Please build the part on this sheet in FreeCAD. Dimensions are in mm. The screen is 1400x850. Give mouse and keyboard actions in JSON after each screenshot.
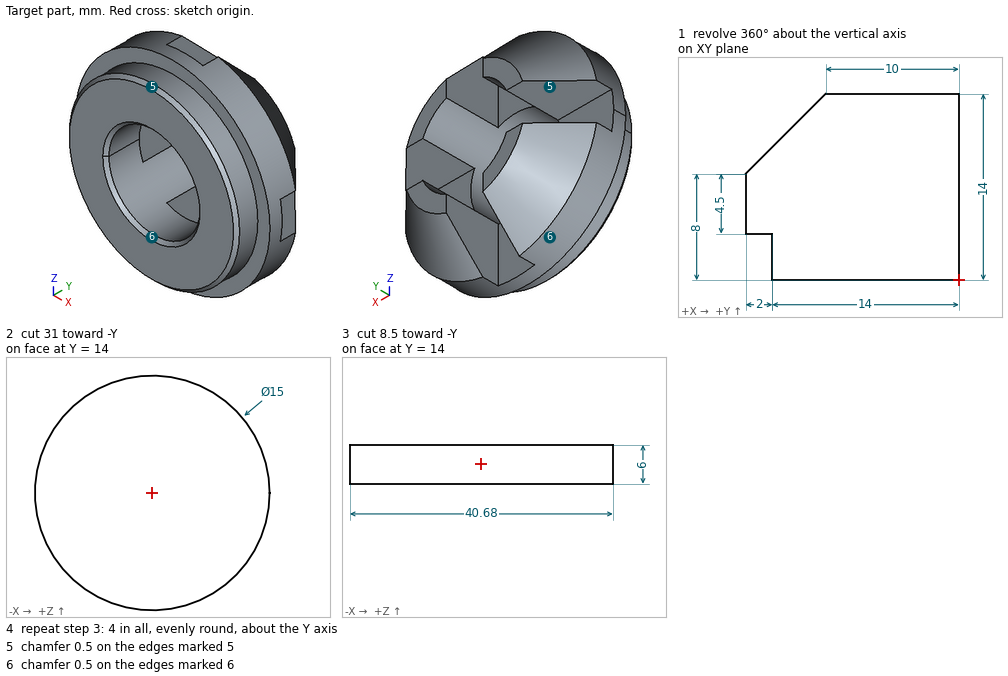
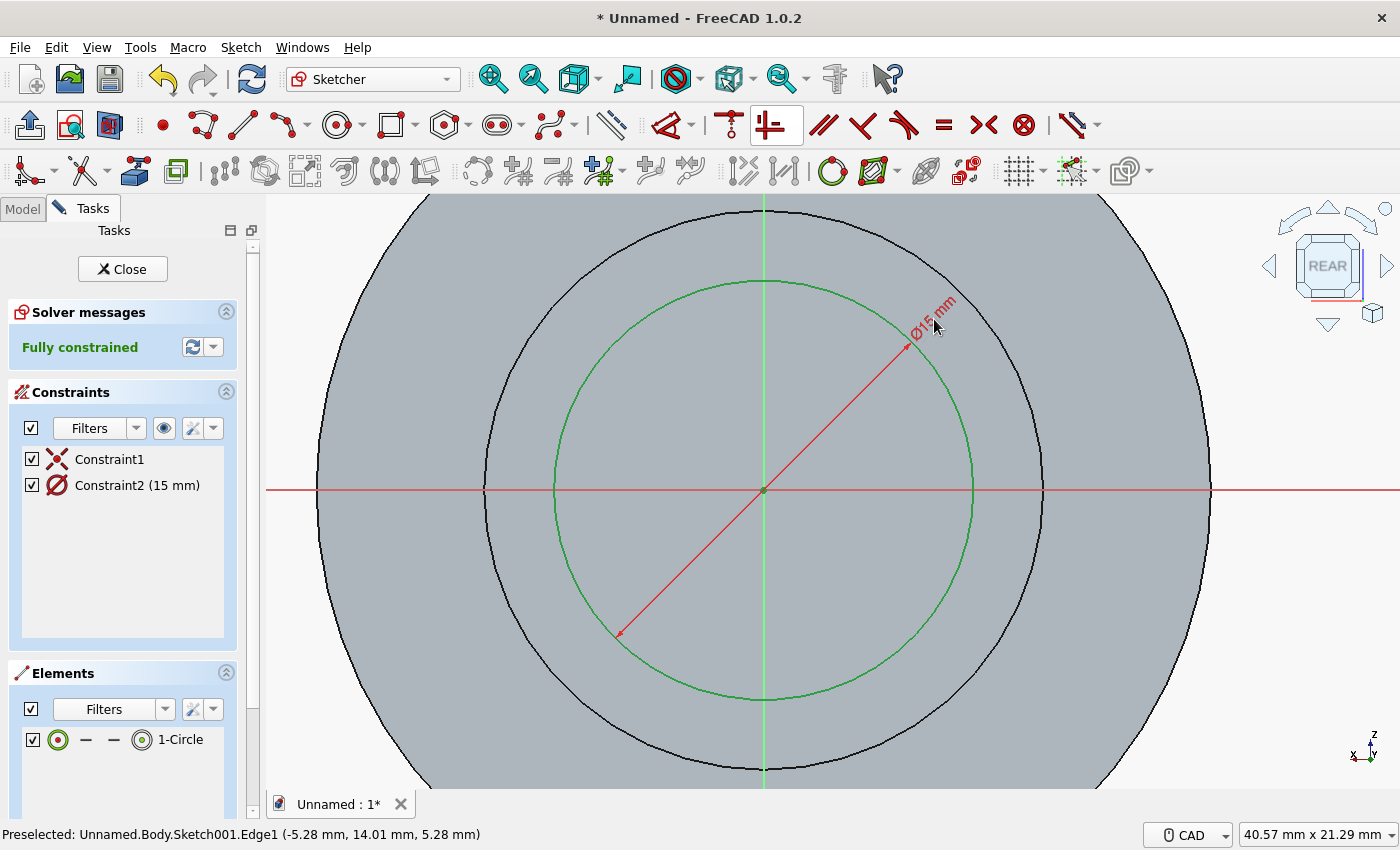
{"action": "left_click", "coordinate": [123, 269]}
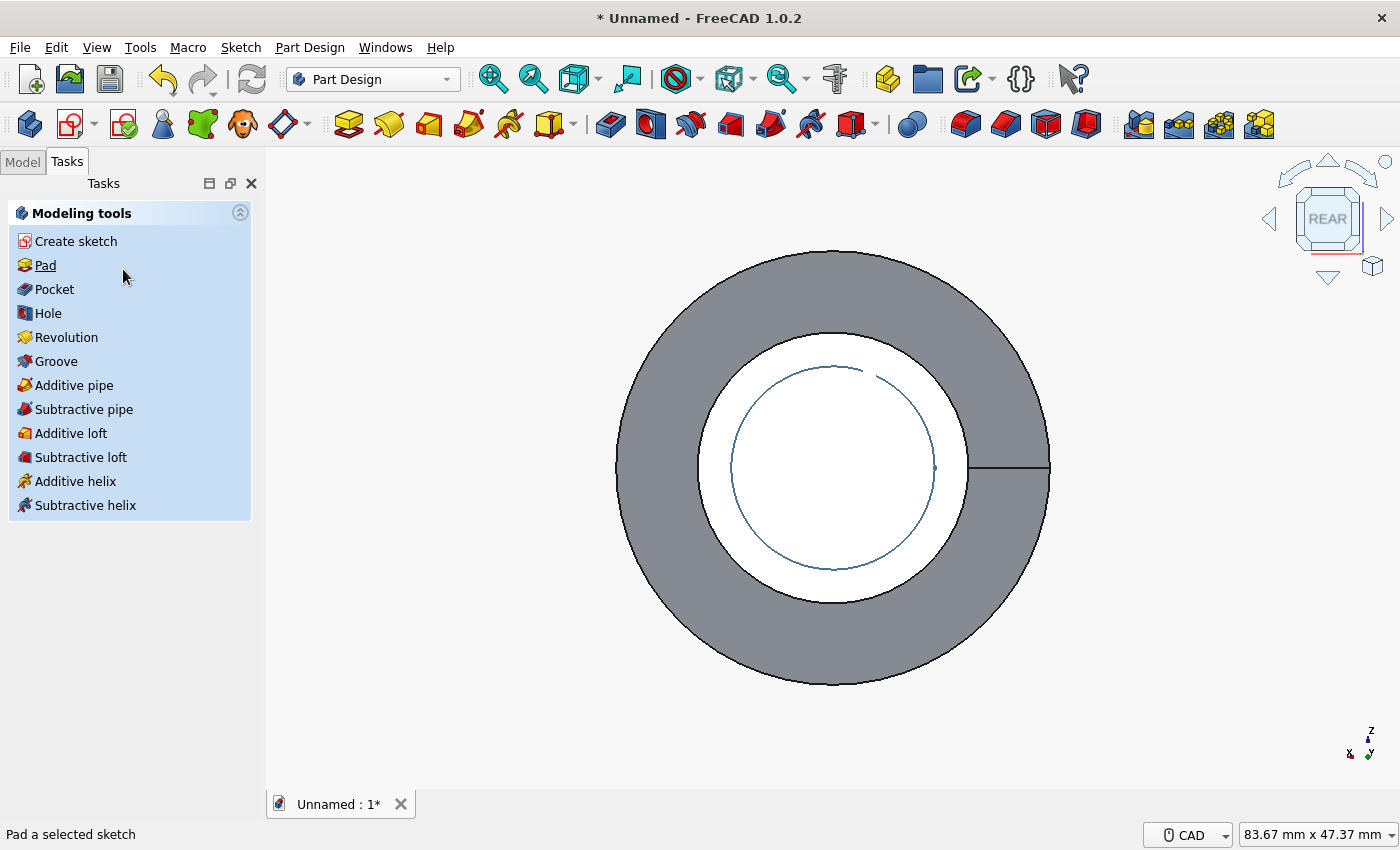
{"action": "left_click", "coordinate": [612, 124]}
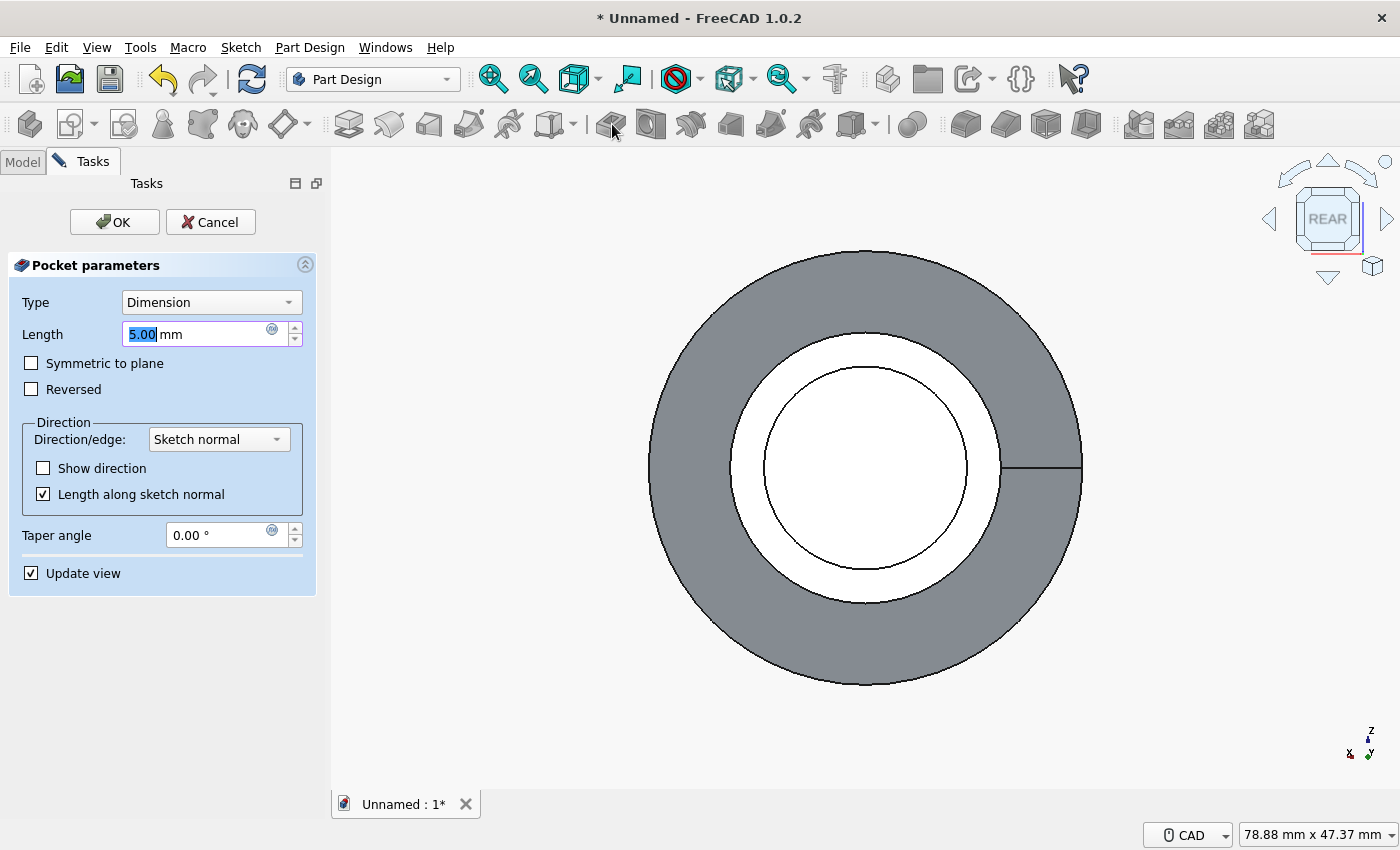
{"action": "type", "text": "31"}
{"action": "key", "text": "Tab"}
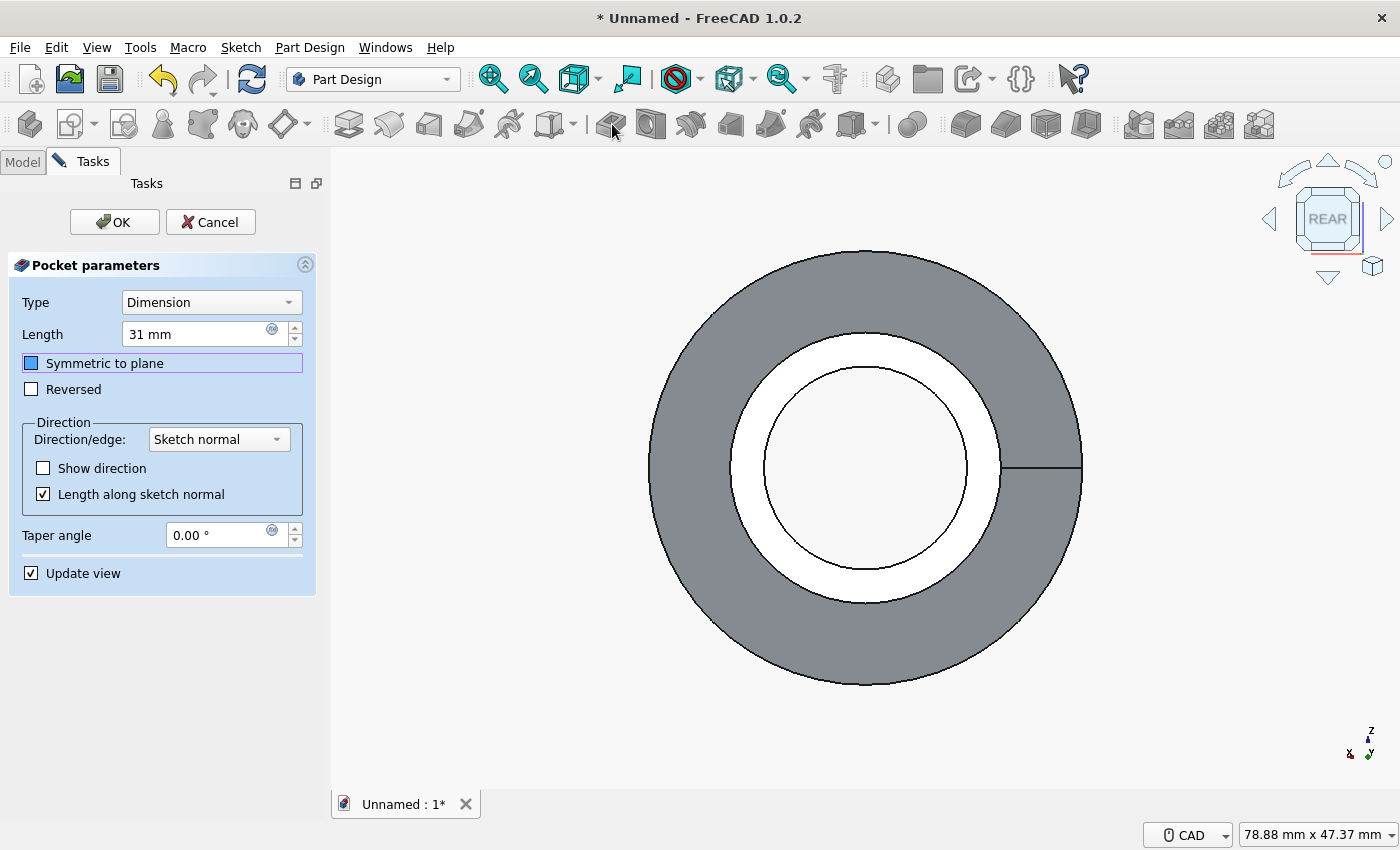
{"action": "left_click", "coordinate": [115, 222]}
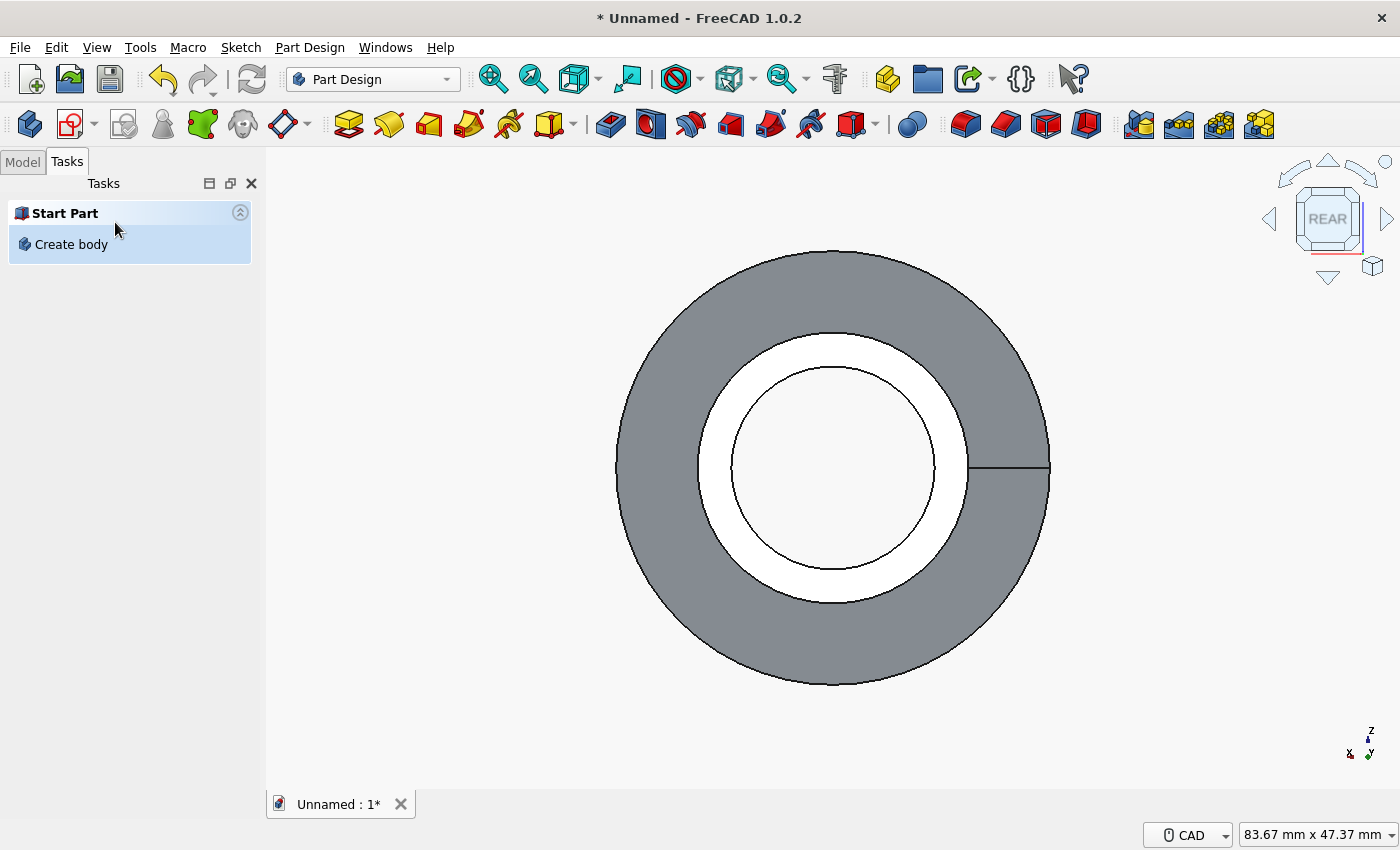
{"action": "left_click", "coordinate": [717, 467]}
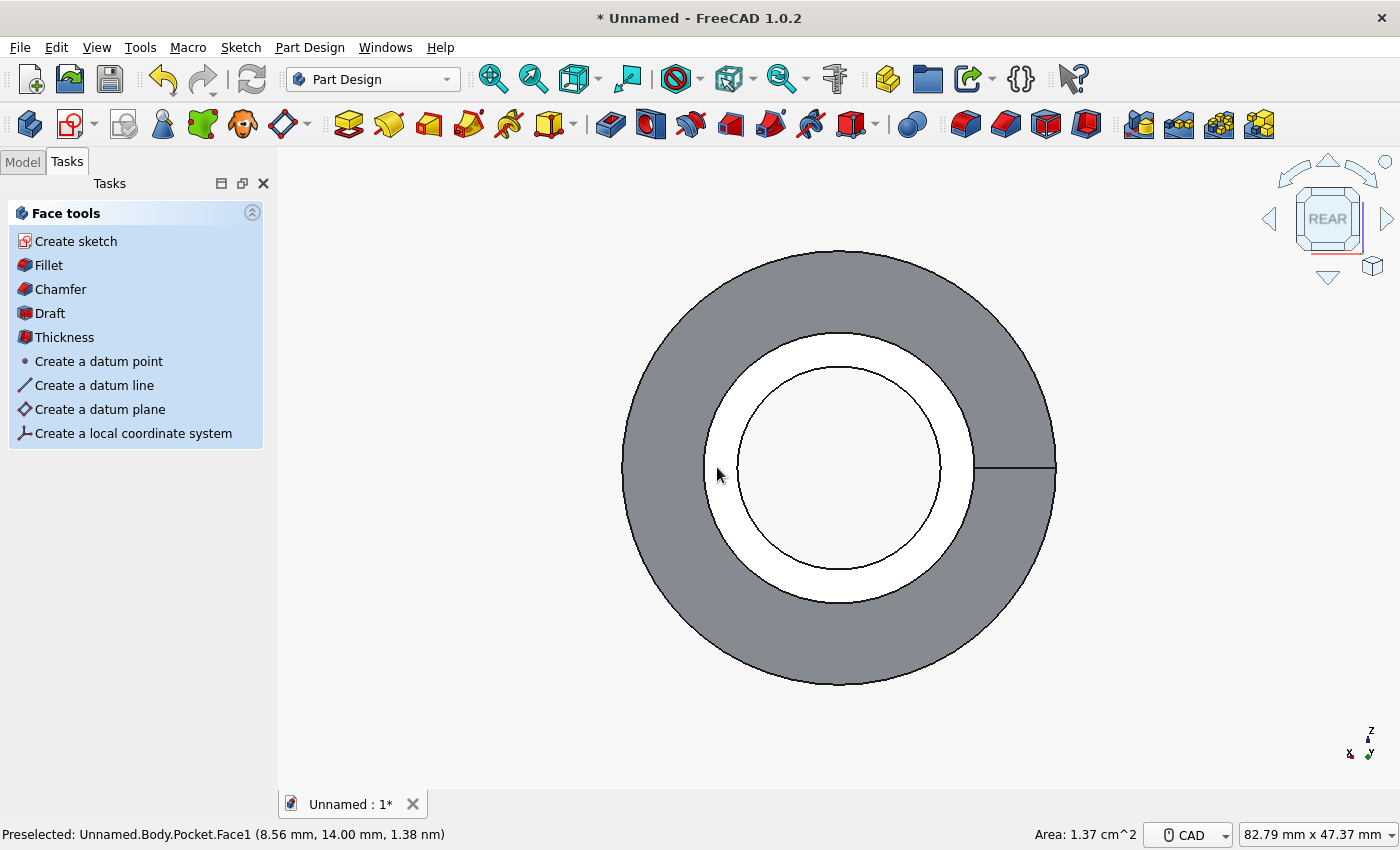
{"action": "left_click", "coordinate": [70, 124]}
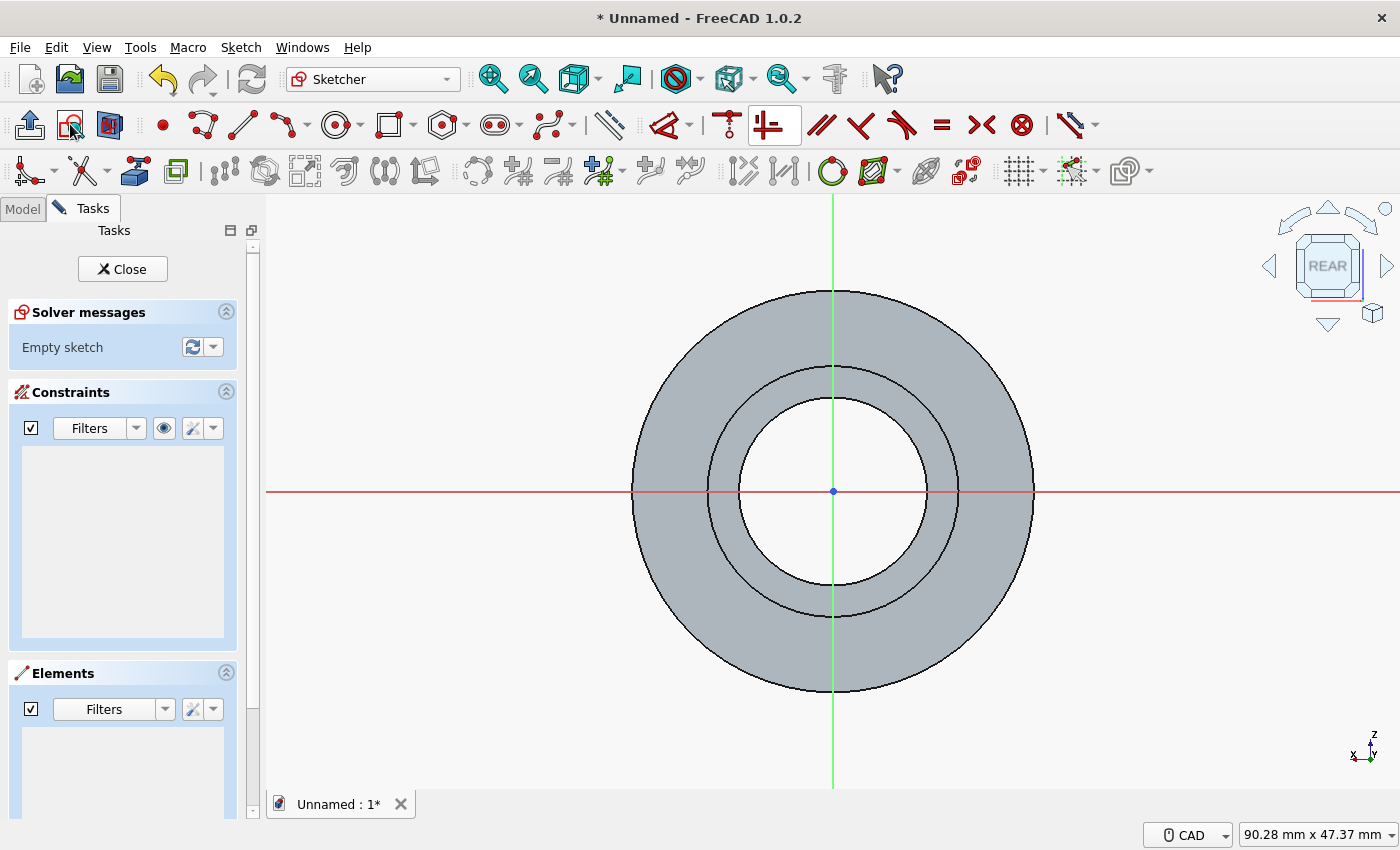
{"action": "left_click", "coordinate": [416, 126]}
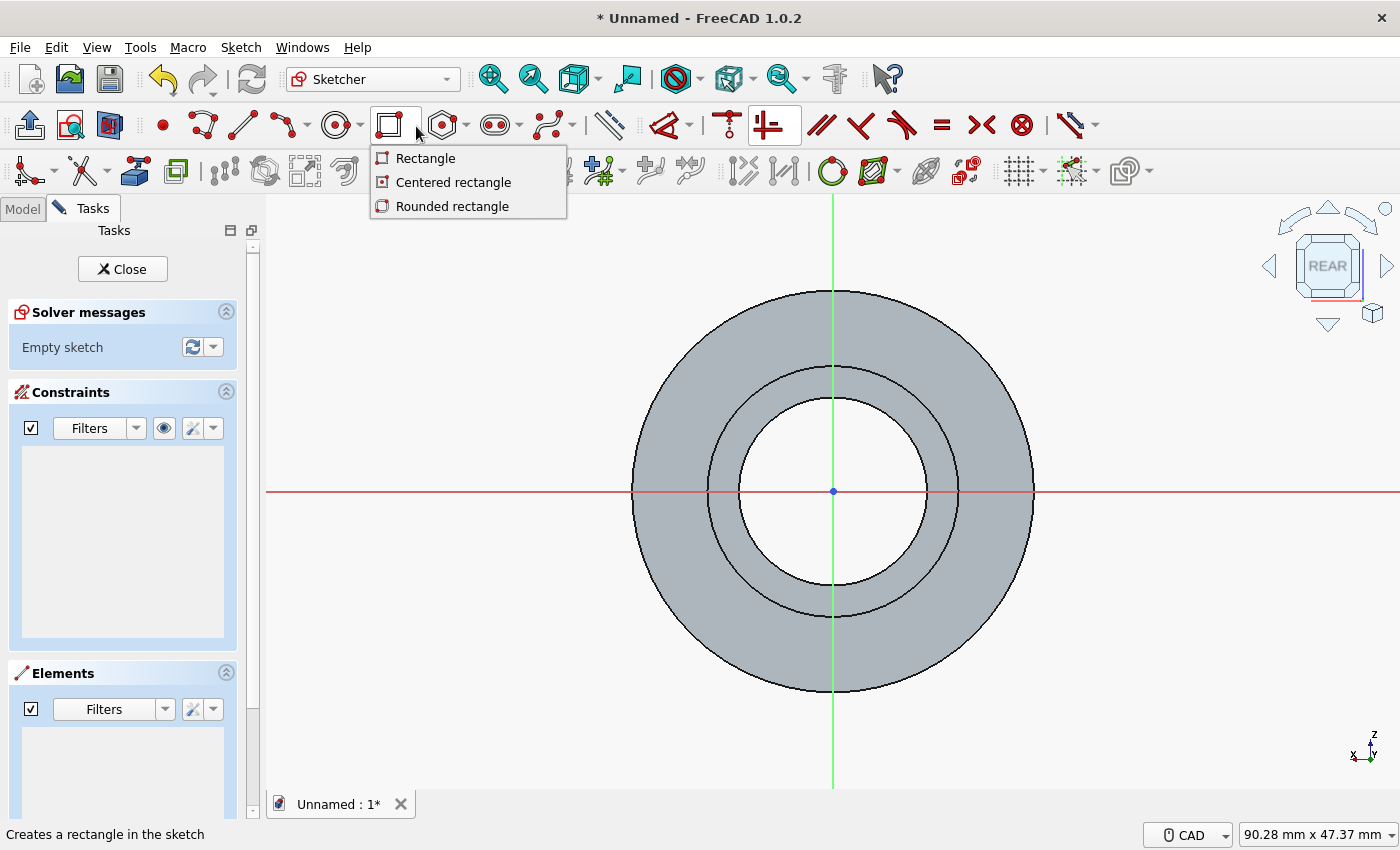
{"action": "left_click", "coordinate": [468, 182]}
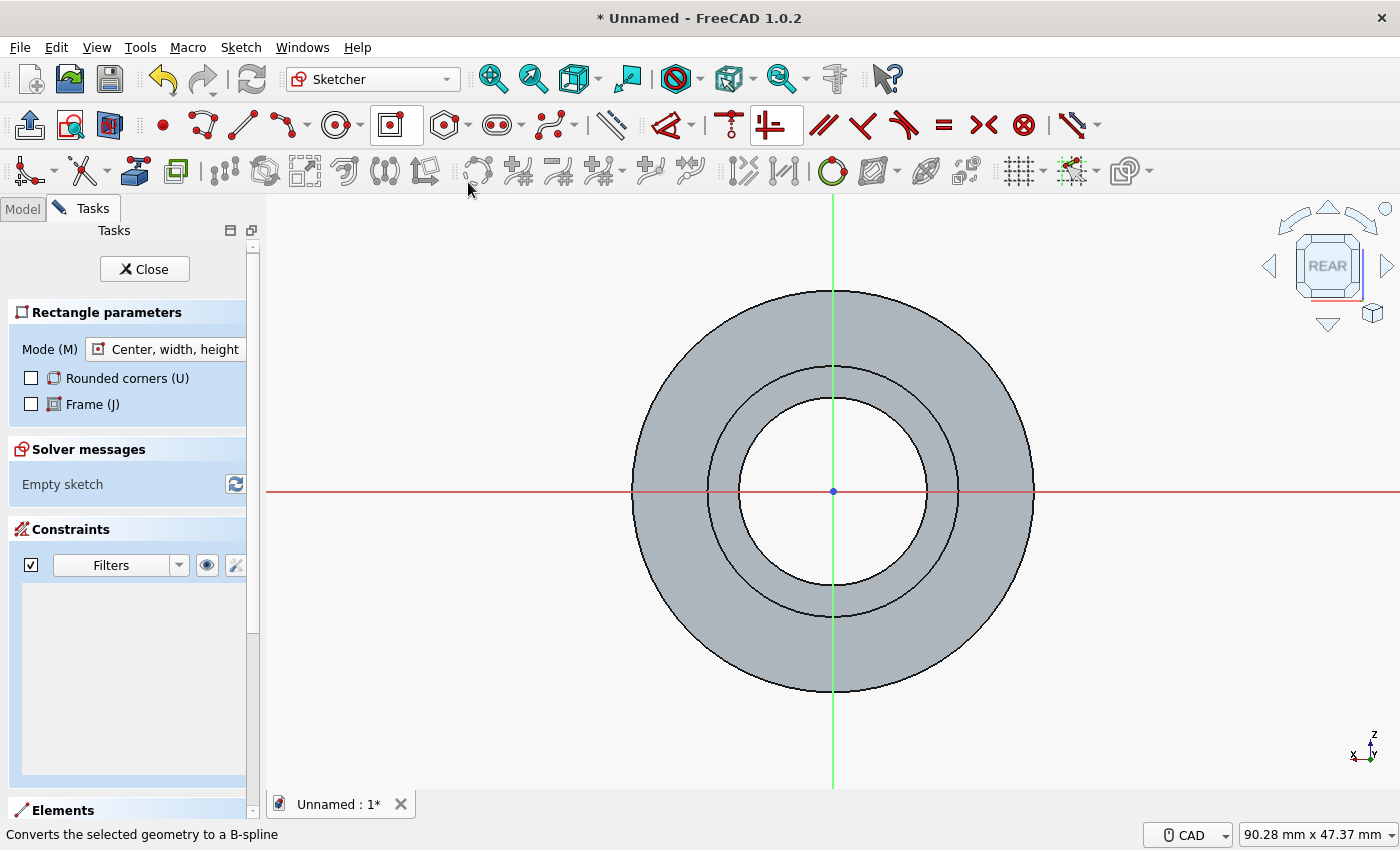
{"action": "left_click", "coordinate": [833, 492]}
{"action": "left_click", "coordinate": [1088, 454]}
{"action": "key", "text": "Escape"}